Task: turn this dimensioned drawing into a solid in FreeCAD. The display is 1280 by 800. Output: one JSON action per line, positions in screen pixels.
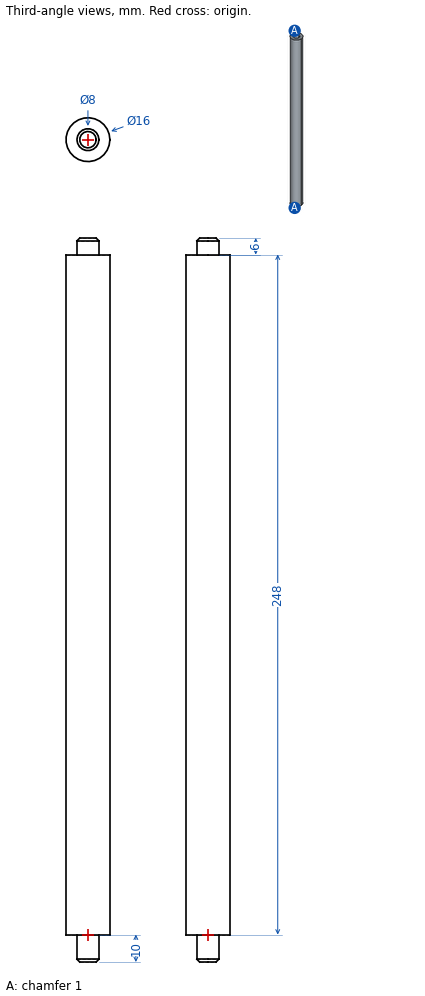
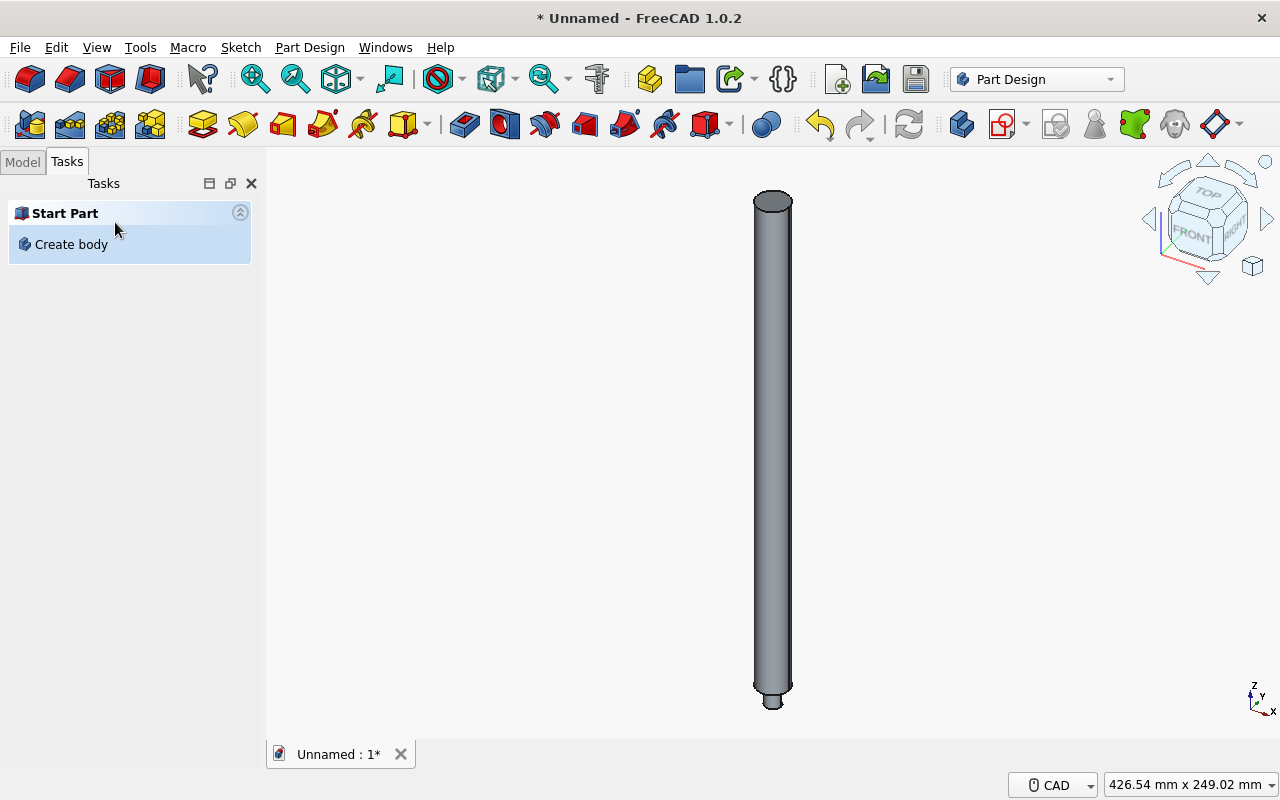
{"action": "left_click", "coordinate": [23, 161]}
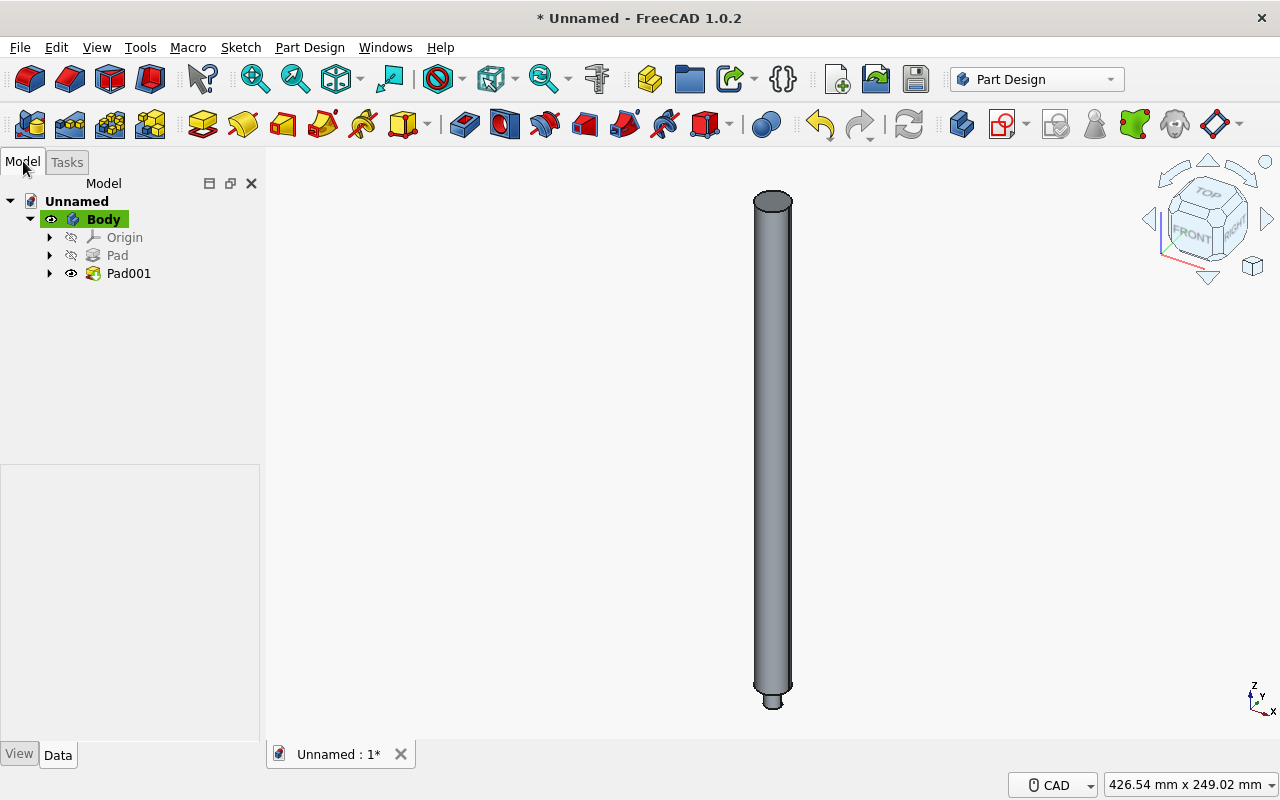
{"action": "left_click", "coordinate": [50, 237]}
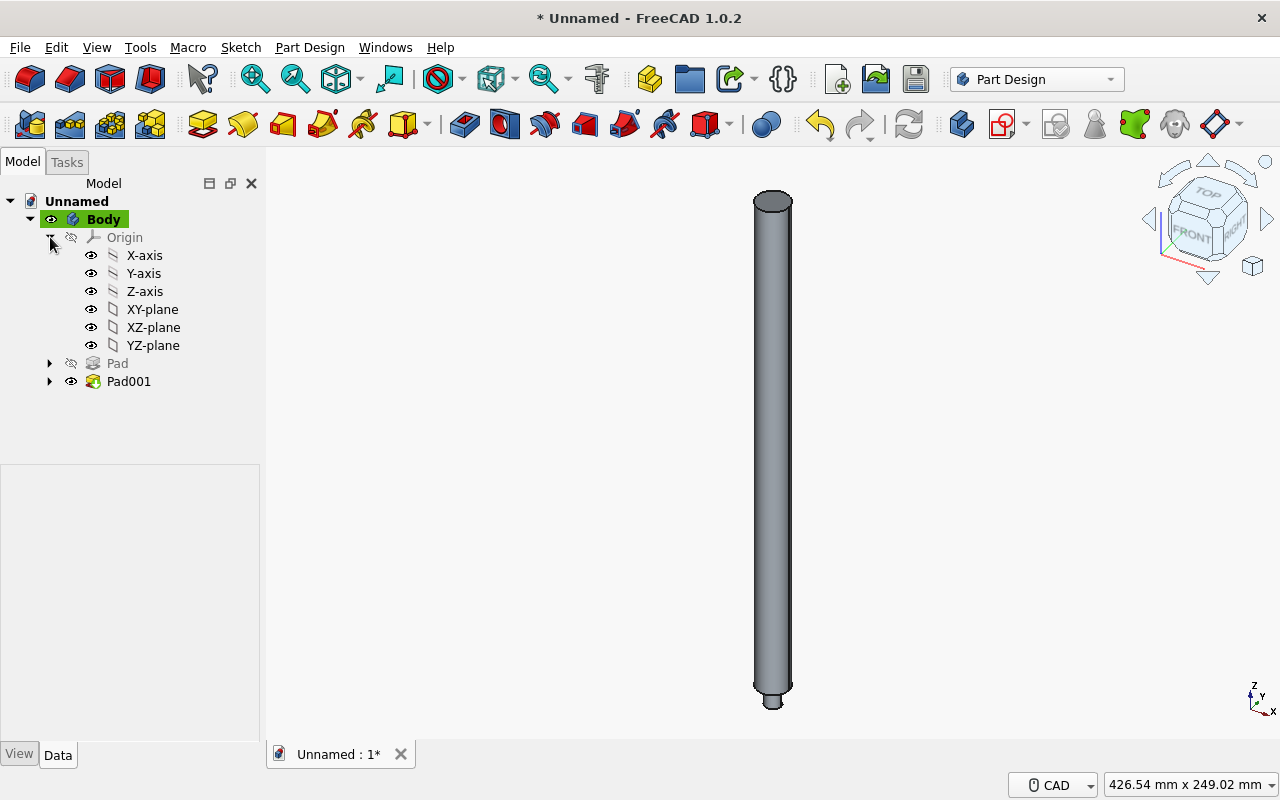
{"action": "left_click", "coordinate": [136, 309]}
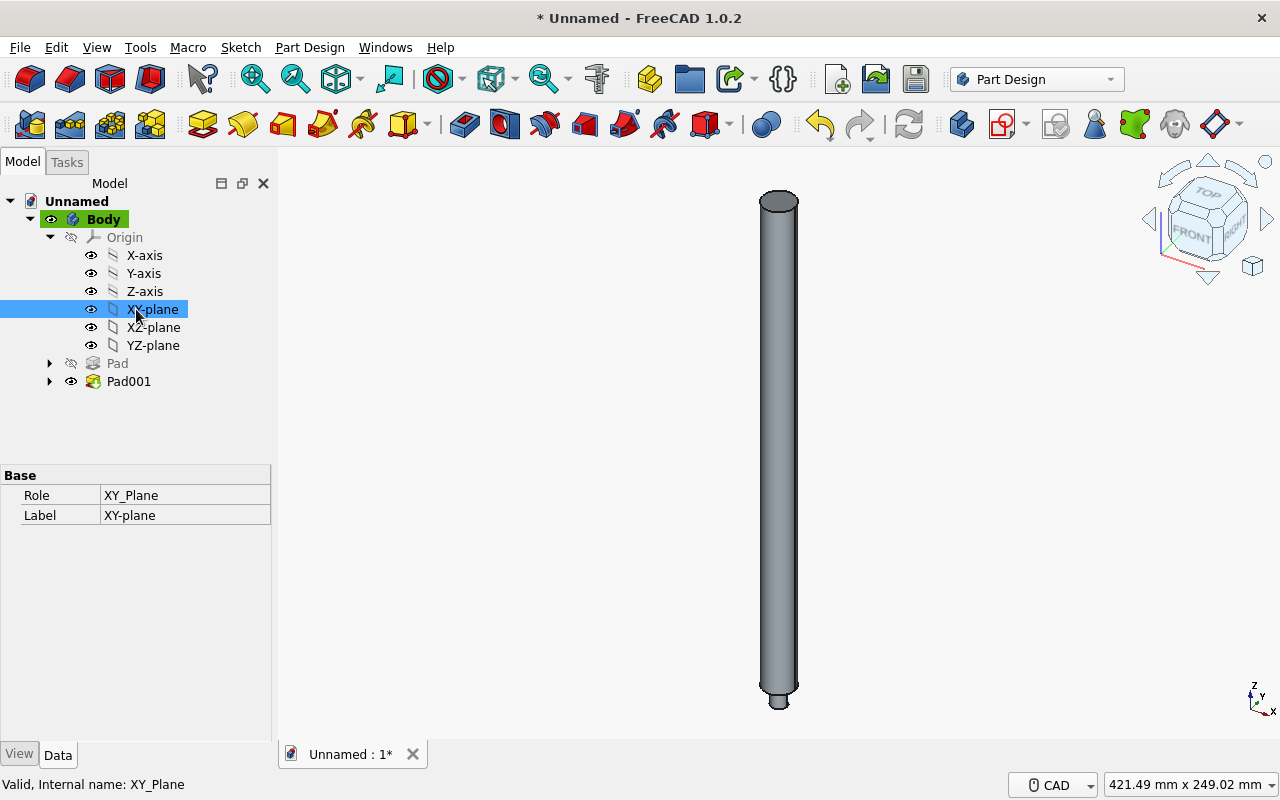
{"action": "left_click", "coordinate": [1216, 124]}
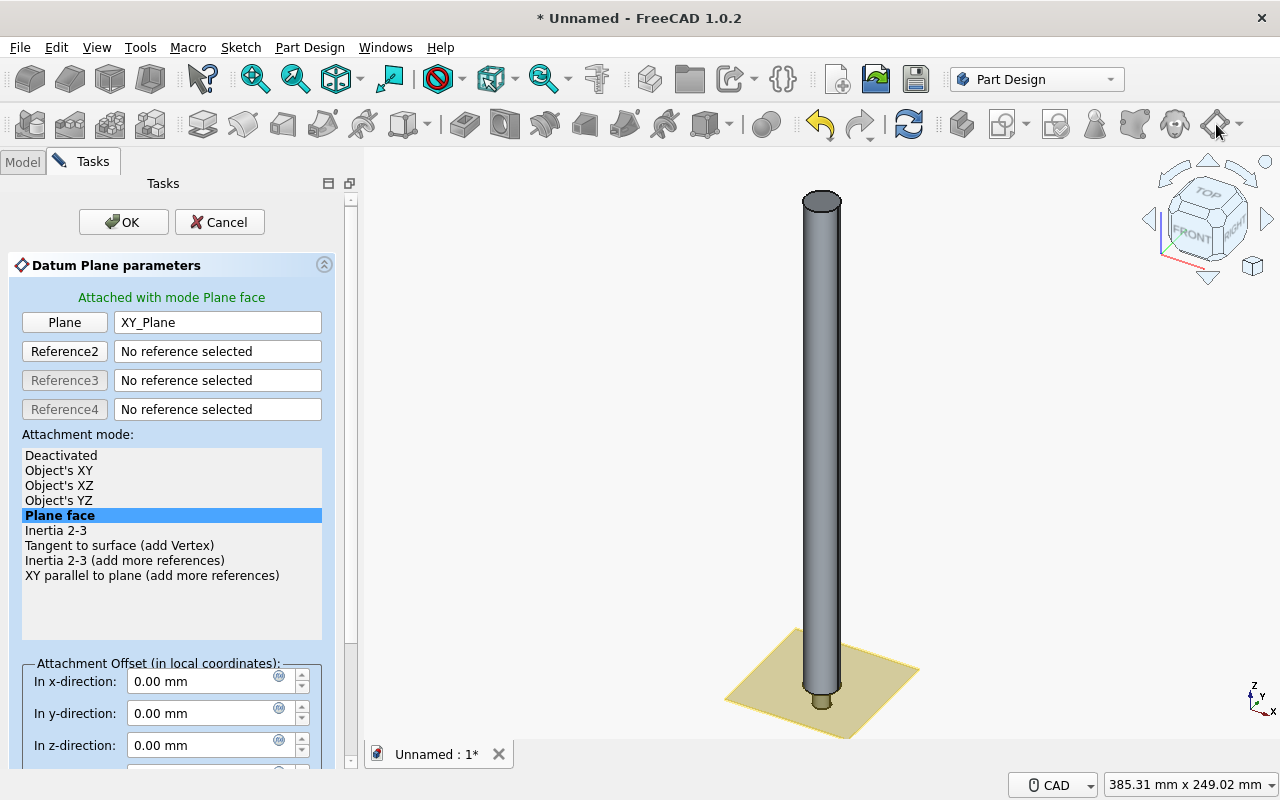
{"action": "triple_click", "coordinate": [210, 745]}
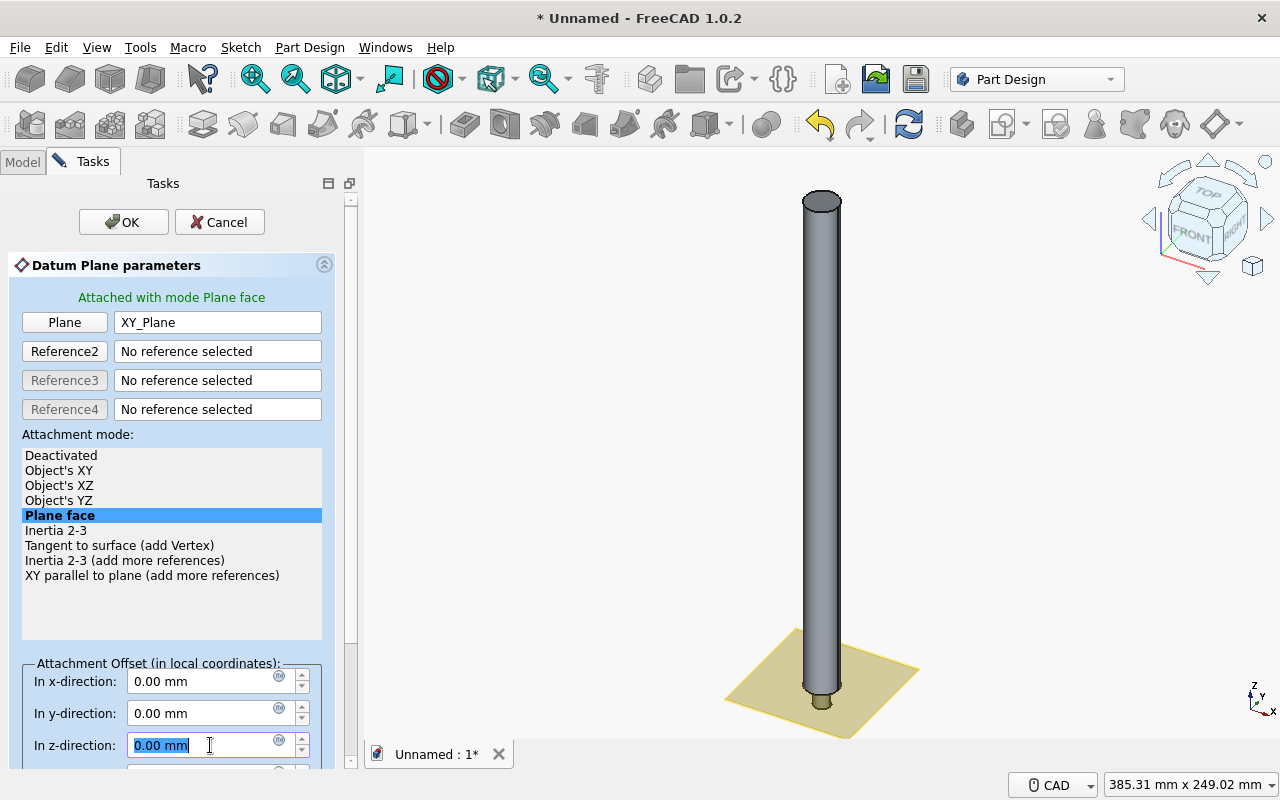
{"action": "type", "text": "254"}
{"action": "key", "text": "Tab"}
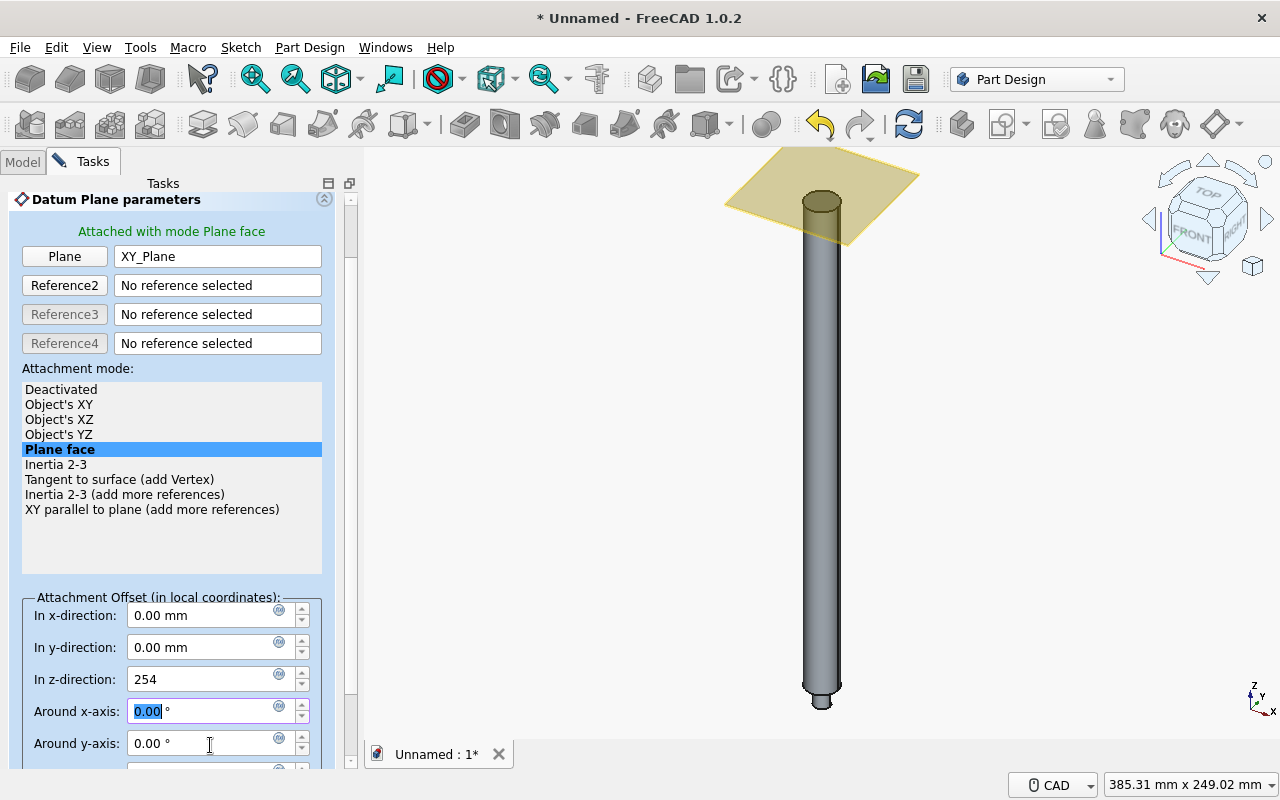
{"action": "scroll", "coordinate": [351, 480], "scroll_direction": "up", "scroll_amount": 2}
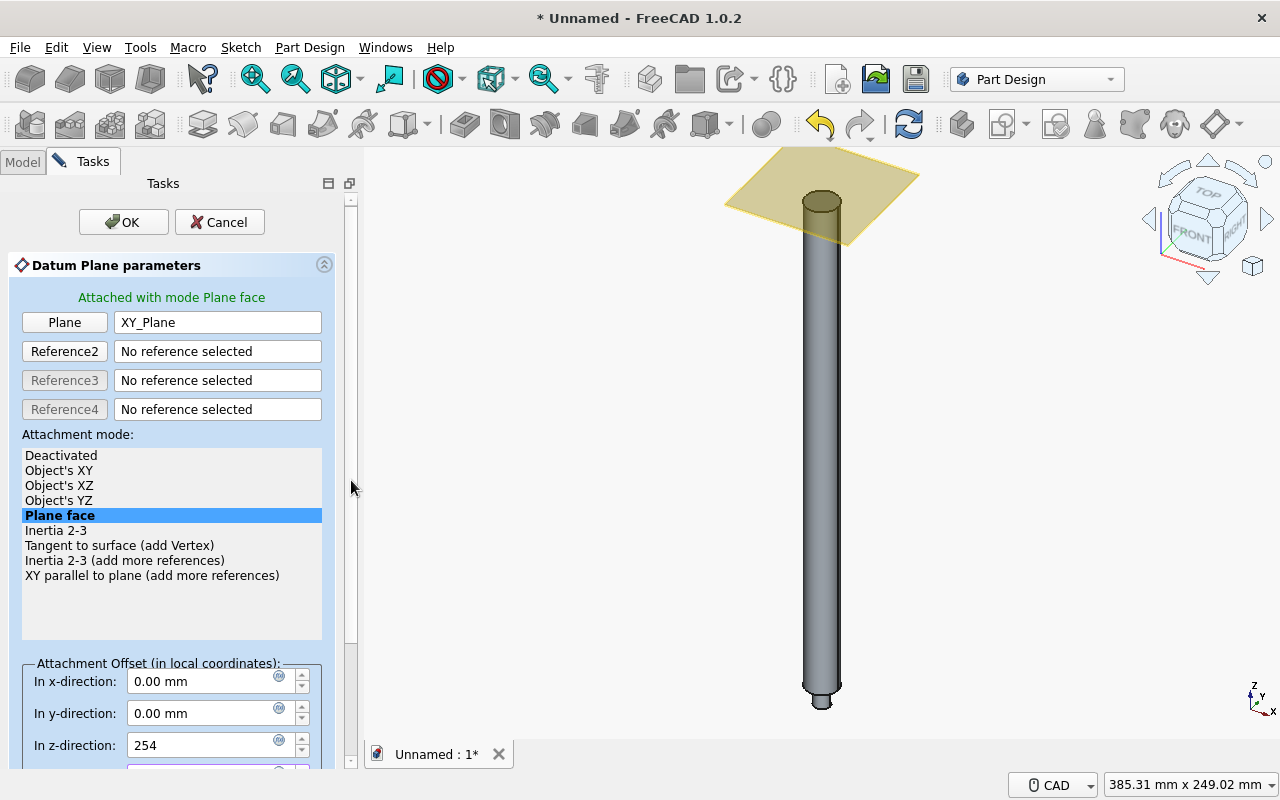
{"action": "left_click", "coordinate": [124, 222]}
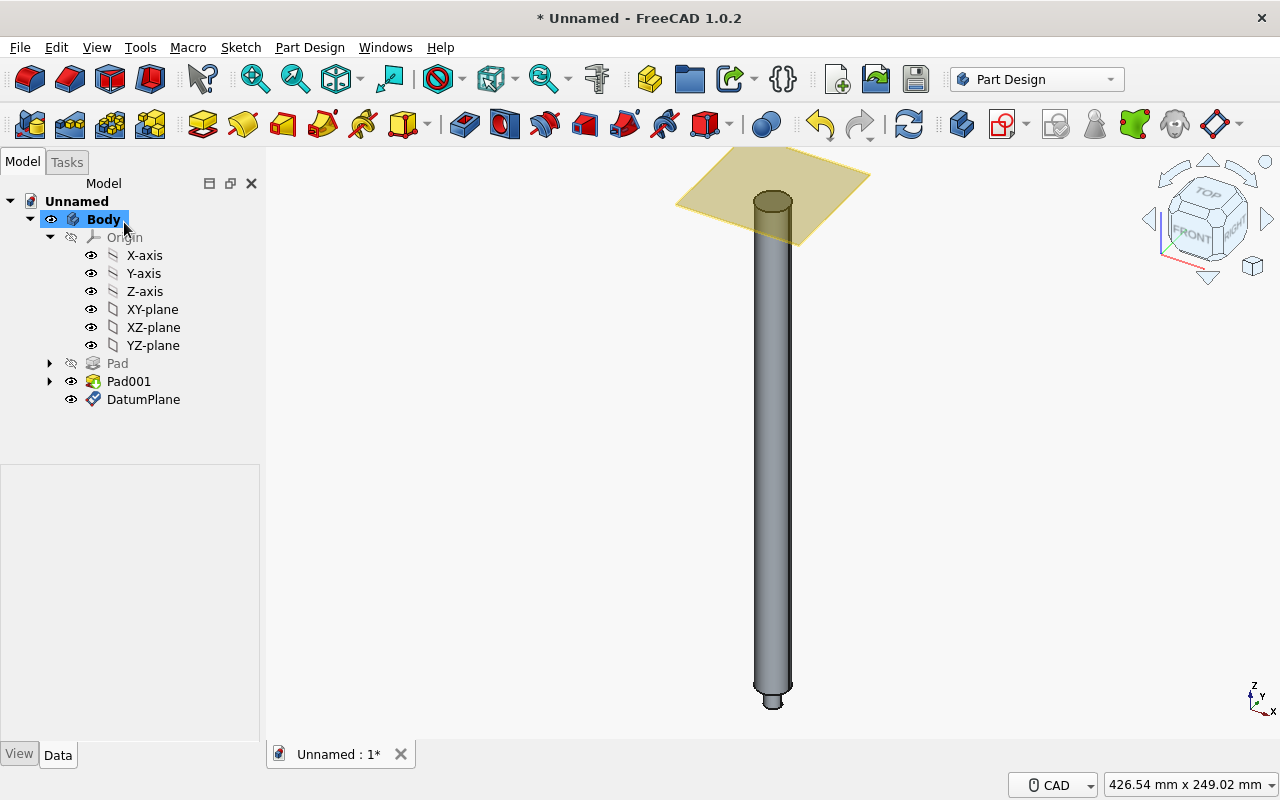
{"action": "left_click", "coordinate": [116, 399]}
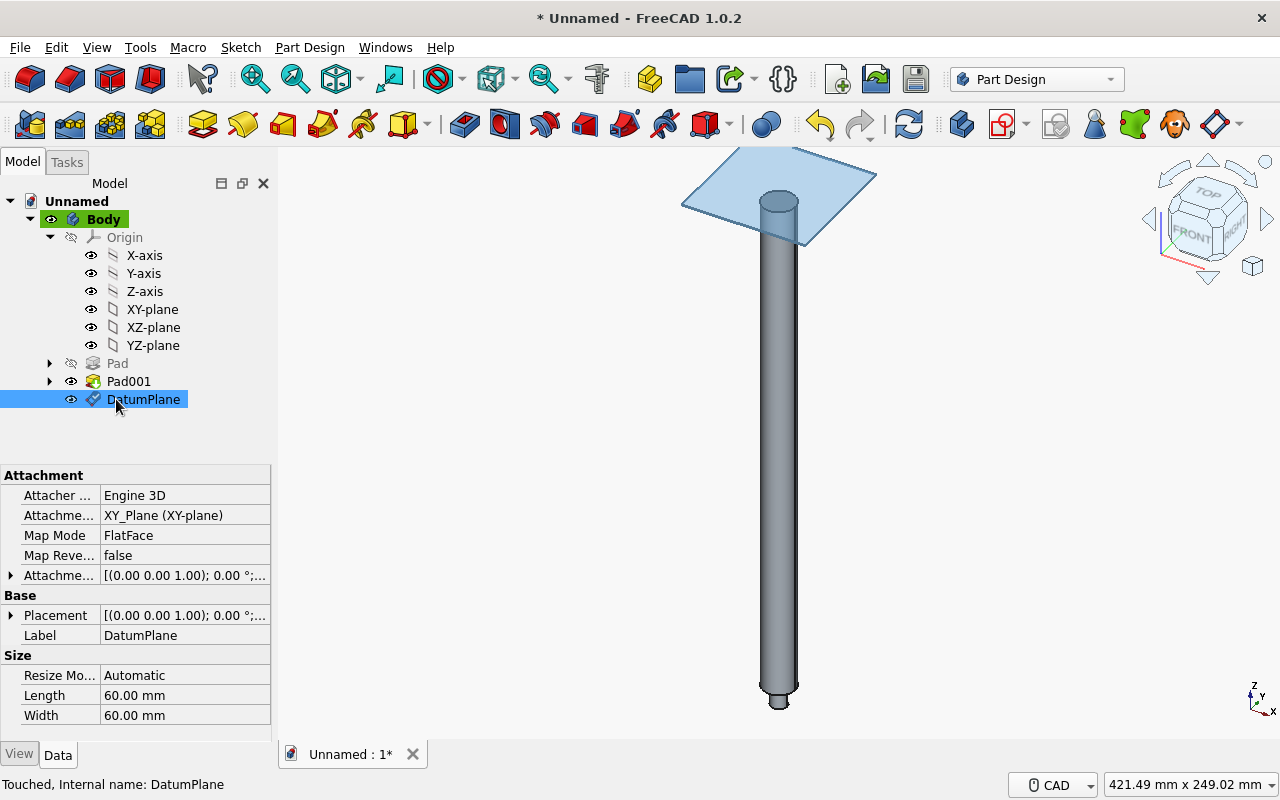
{"action": "left_click", "coordinate": [1002, 124]}